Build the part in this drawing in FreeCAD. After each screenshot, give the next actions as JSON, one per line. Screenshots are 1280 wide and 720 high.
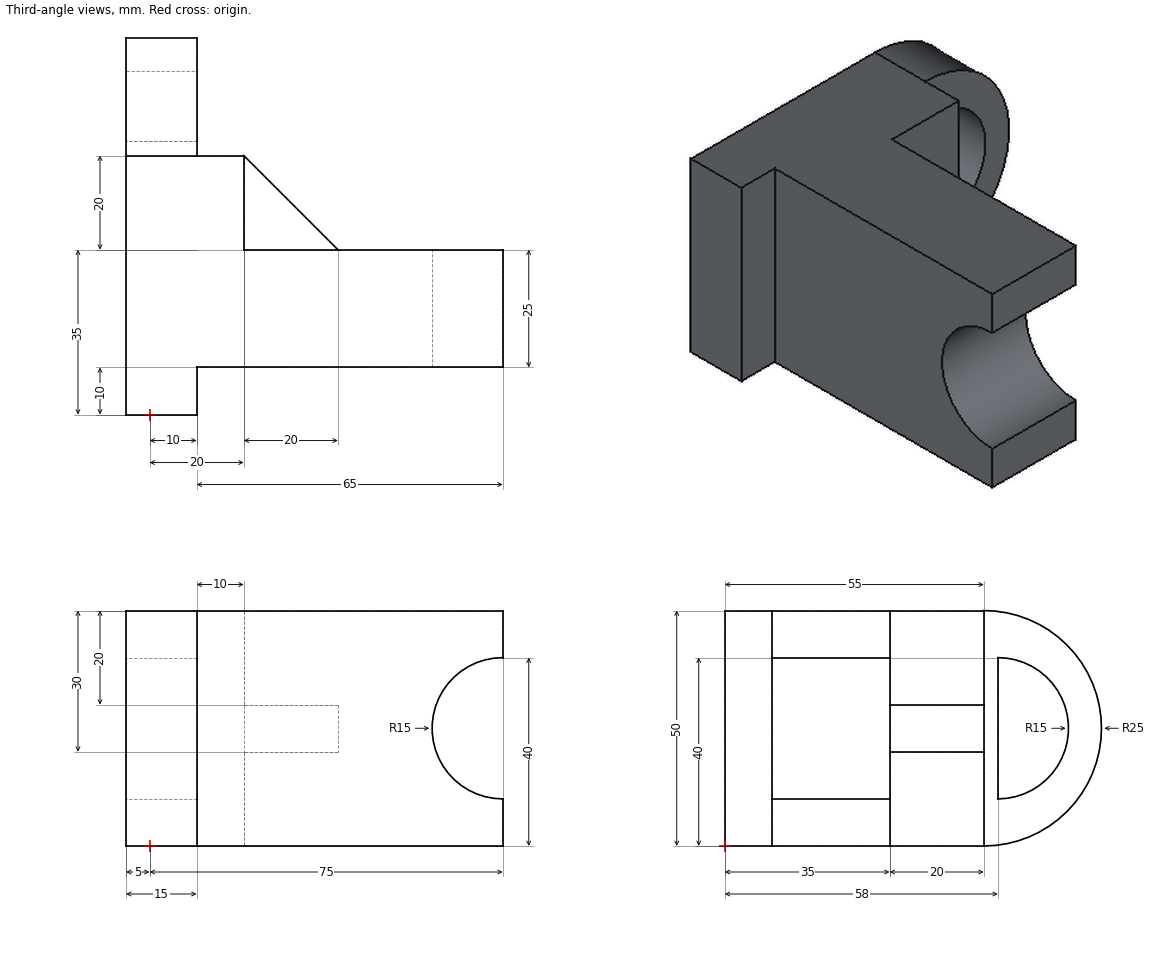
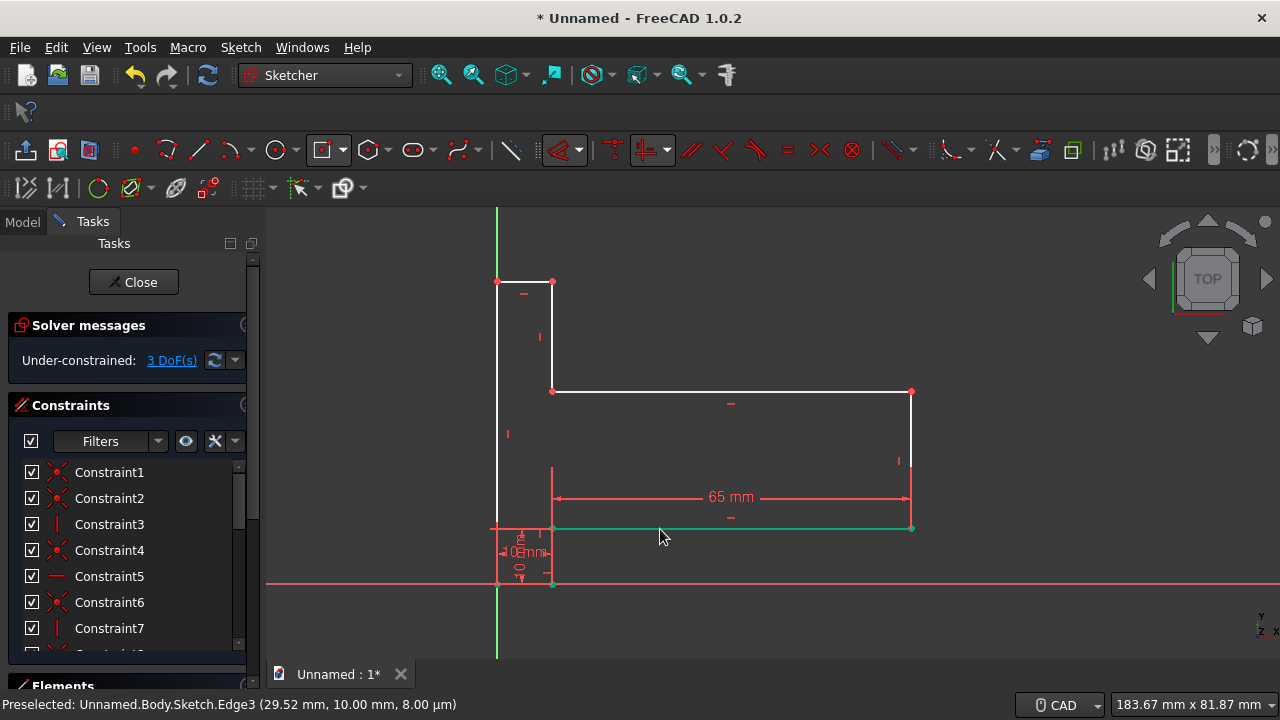
{"action": "left_click", "coordinate": [911, 488]}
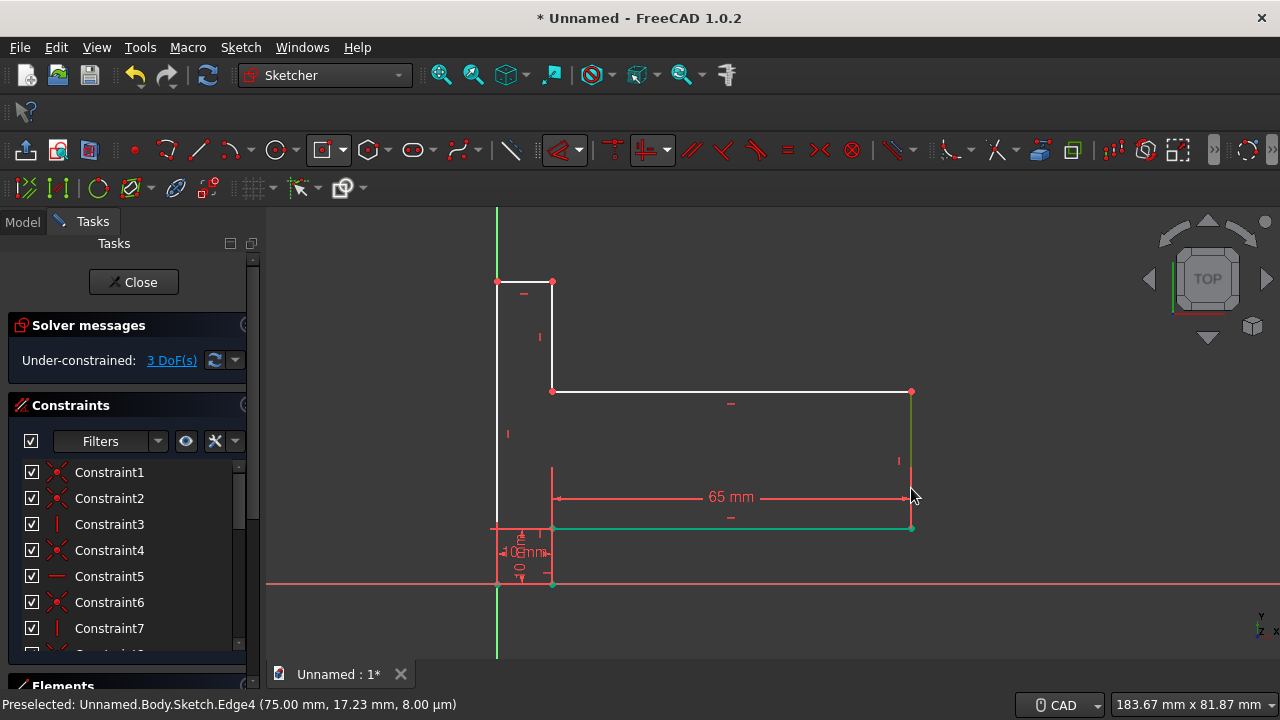
{"action": "key", "text": "i"}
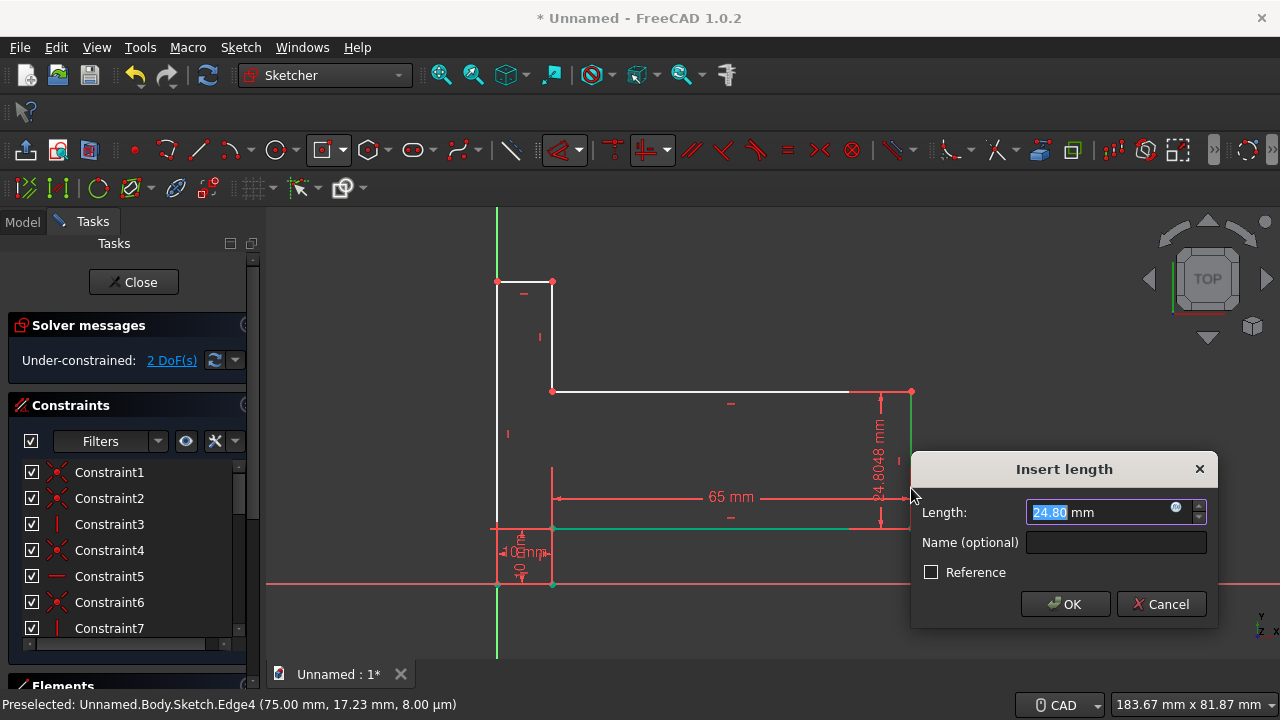
{"action": "type", "text": "25"}
{"action": "key", "text": "Return"}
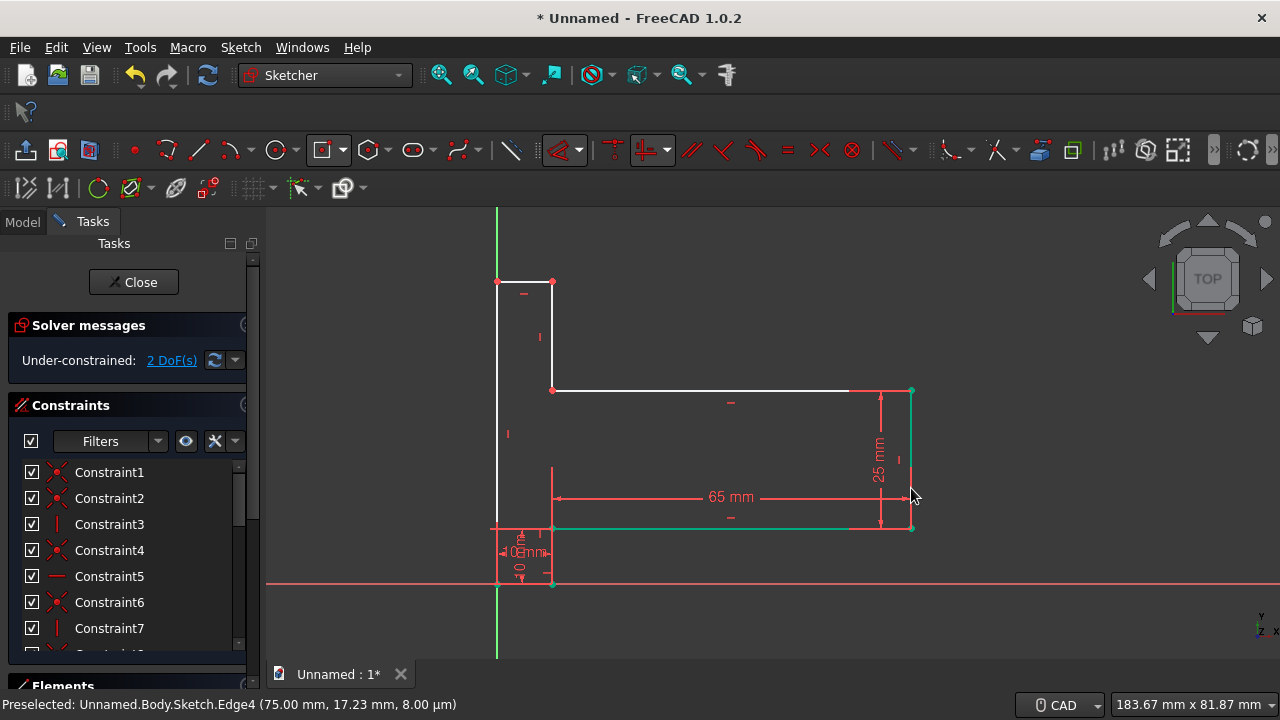
{"action": "left_click", "coordinate": [803, 391]}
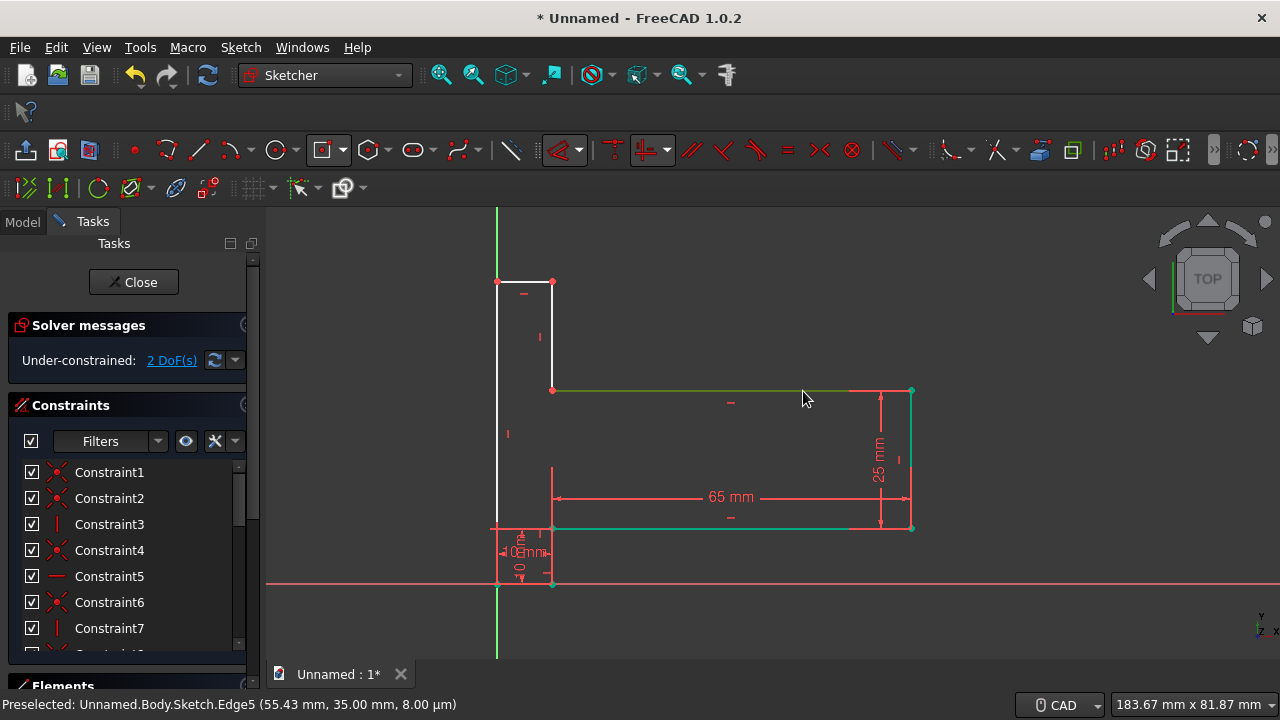
{"action": "left_click", "coordinate": [582, 150]}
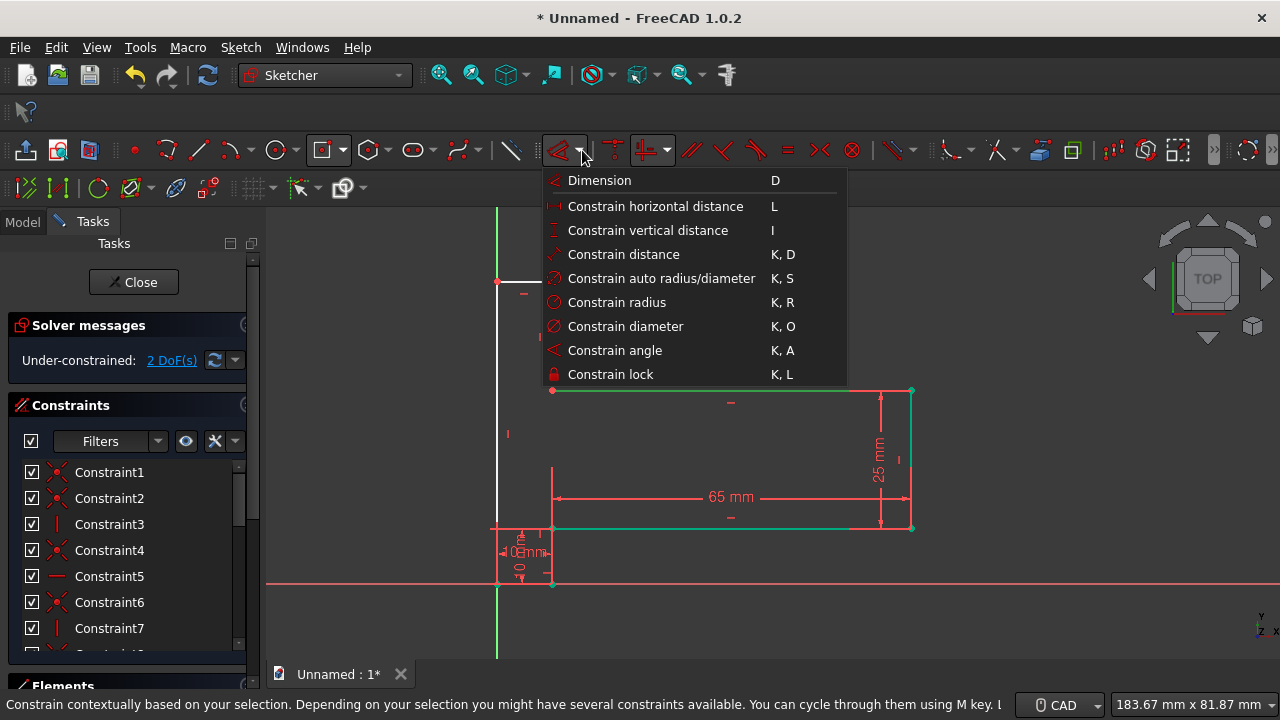
{"action": "left_click", "coordinate": [695, 206]}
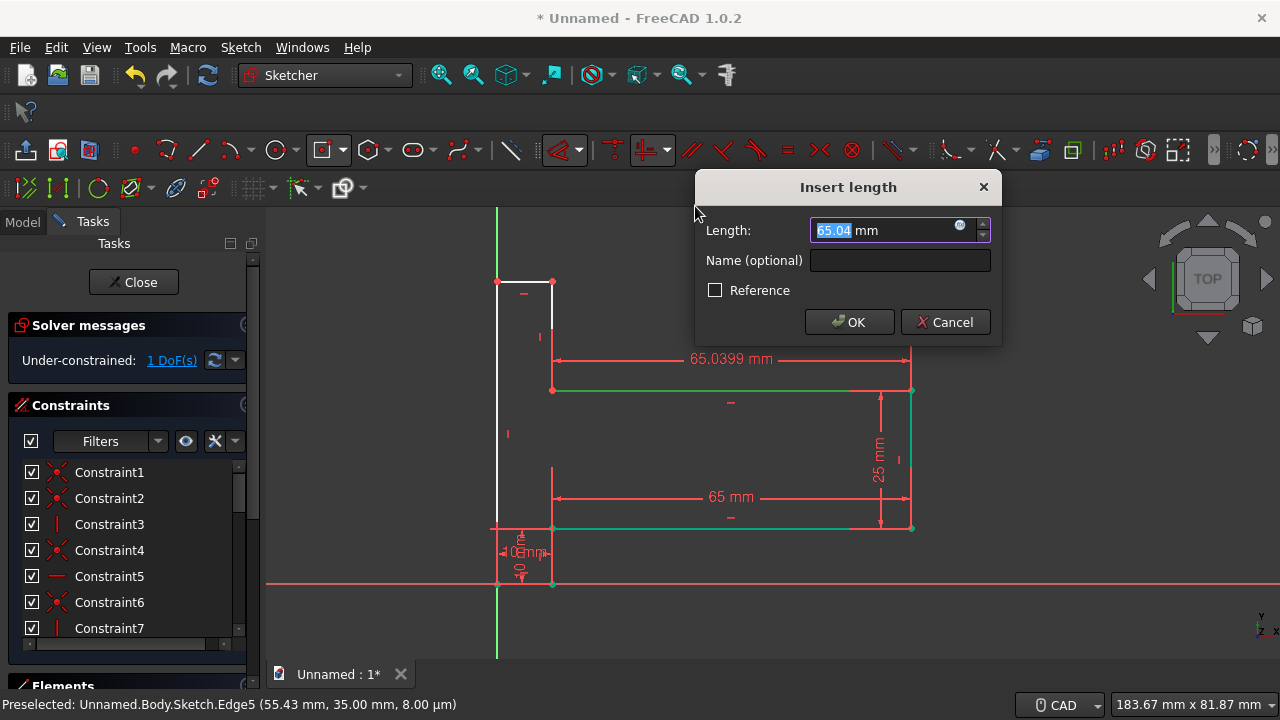
{"action": "type", "text": "65"}
{"action": "key", "text": "Return"}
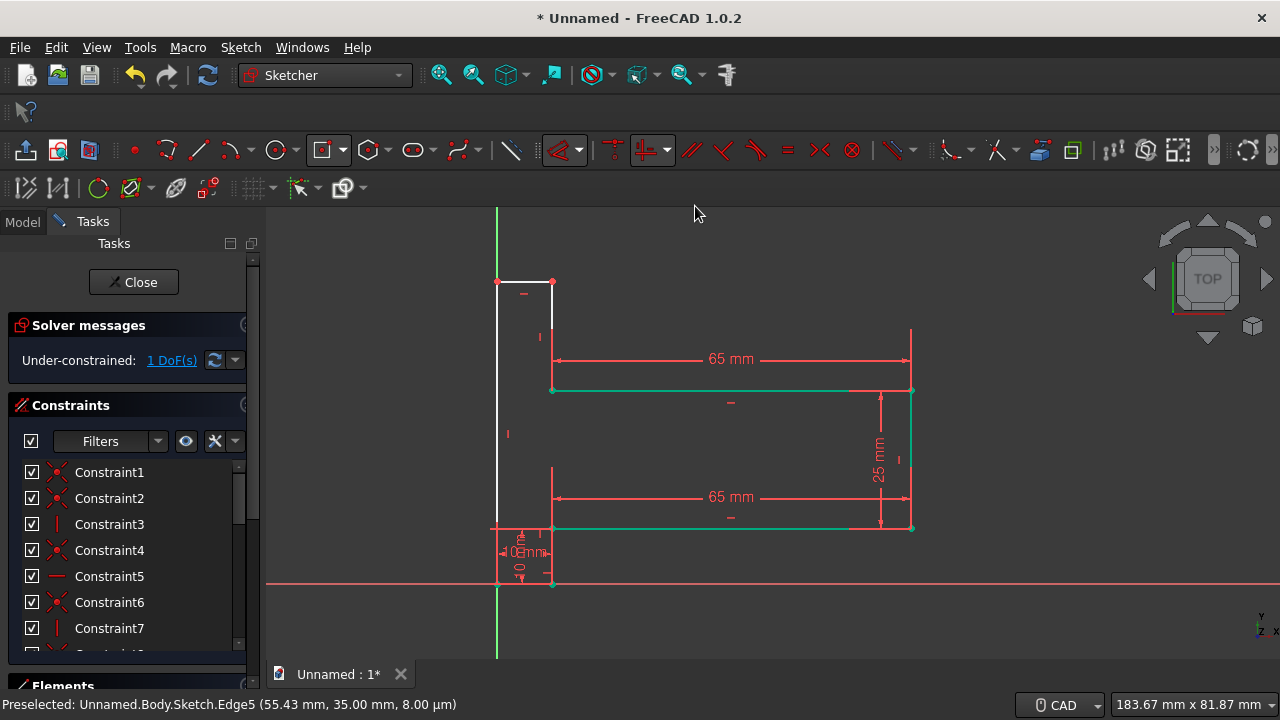
{"action": "left_click", "coordinate": [552, 358]}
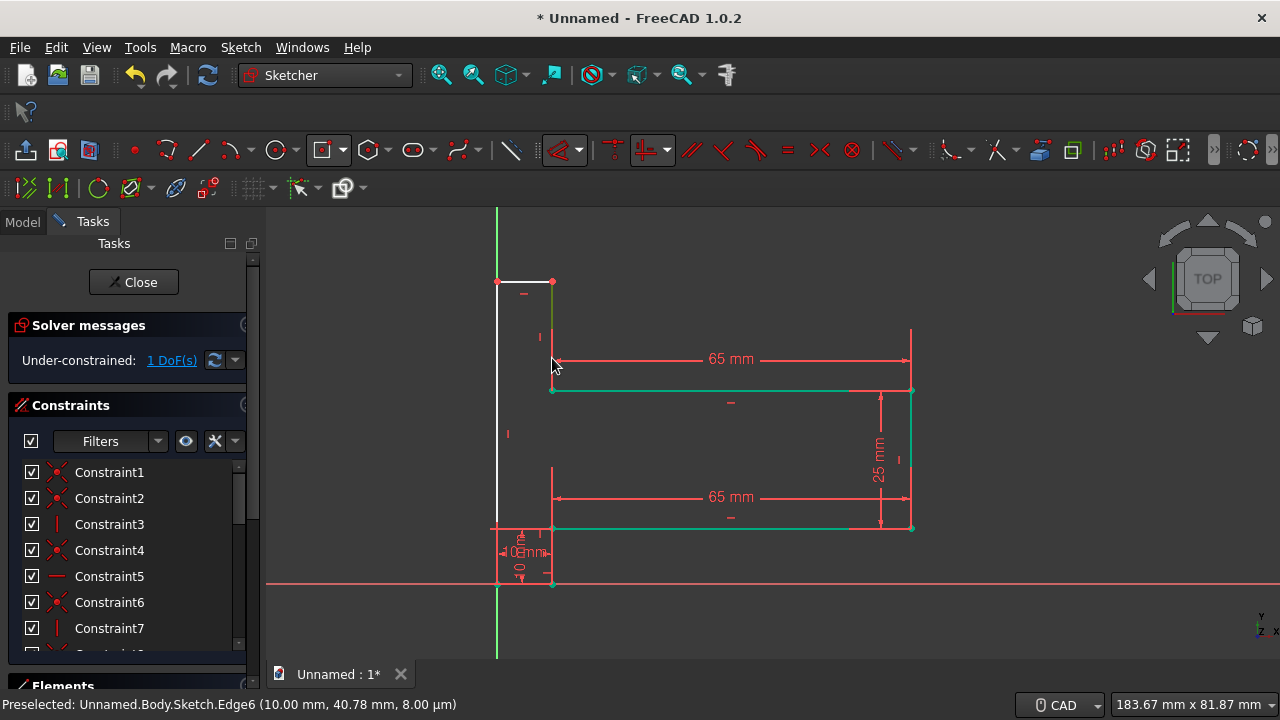
{"action": "key", "text": "i"}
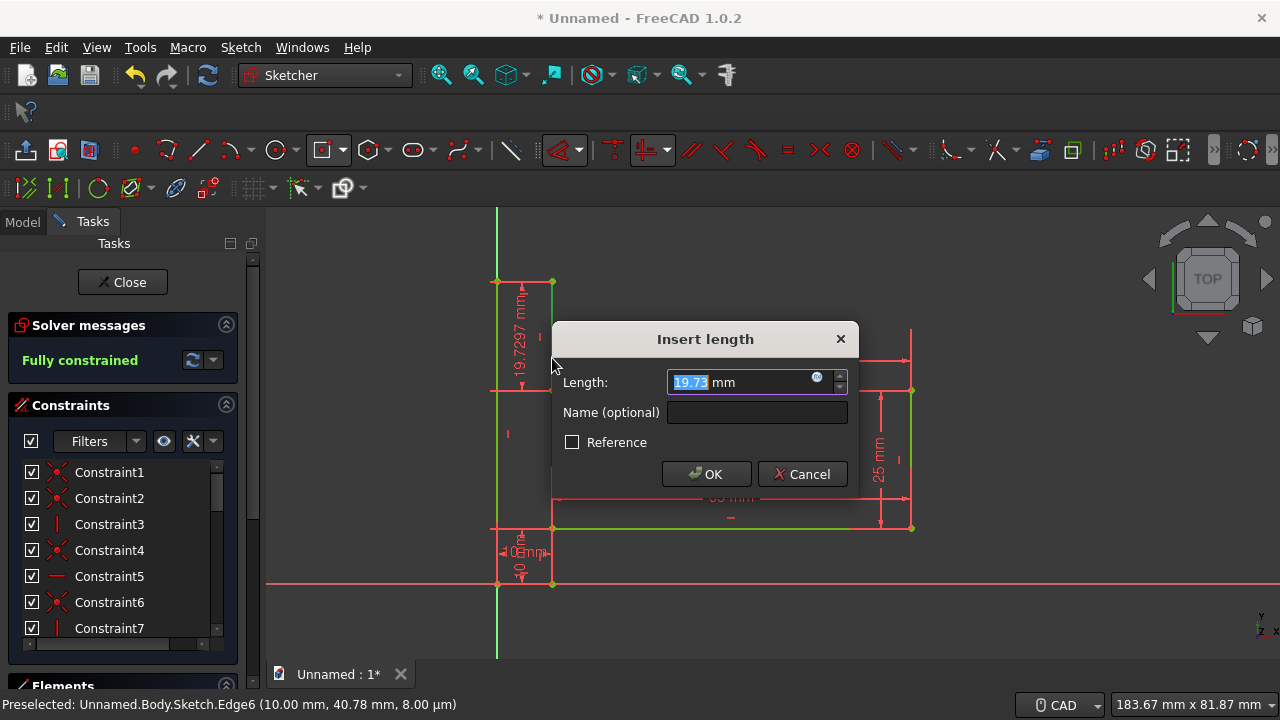
{"action": "type", "text": "20"}
{"action": "key", "text": "Return"}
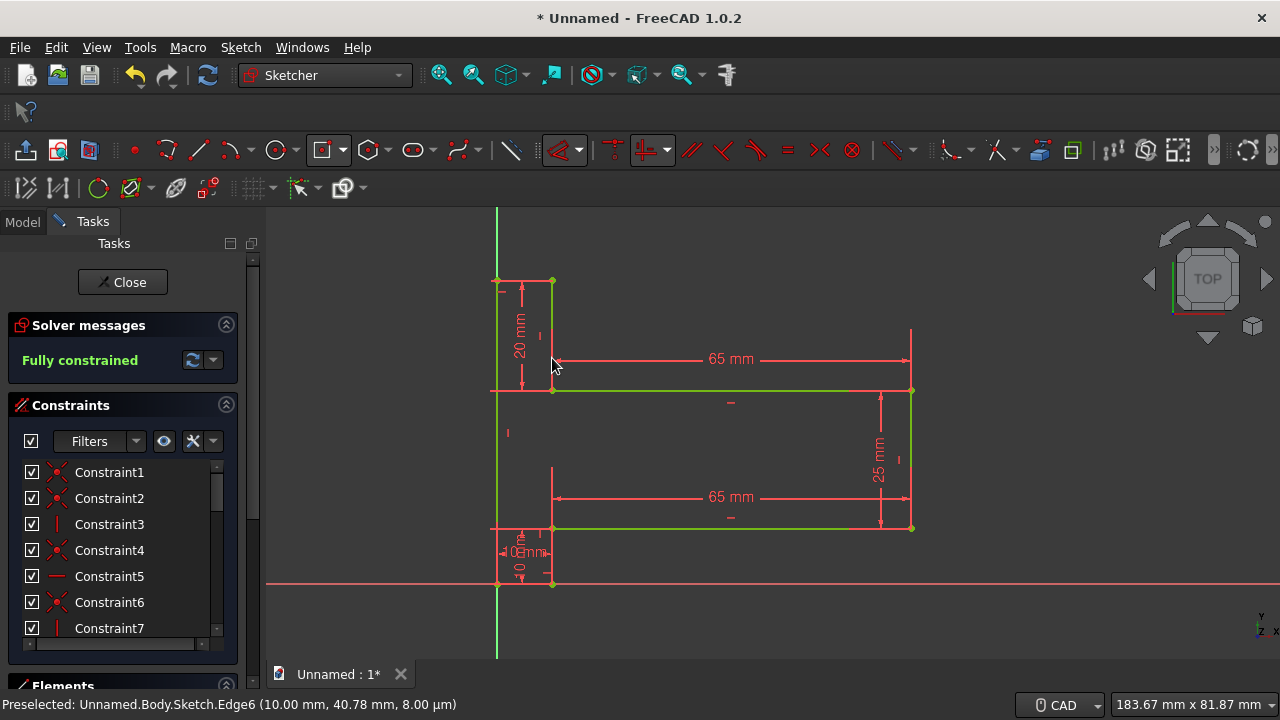
{"action": "left_click", "coordinate": [123, 282]}